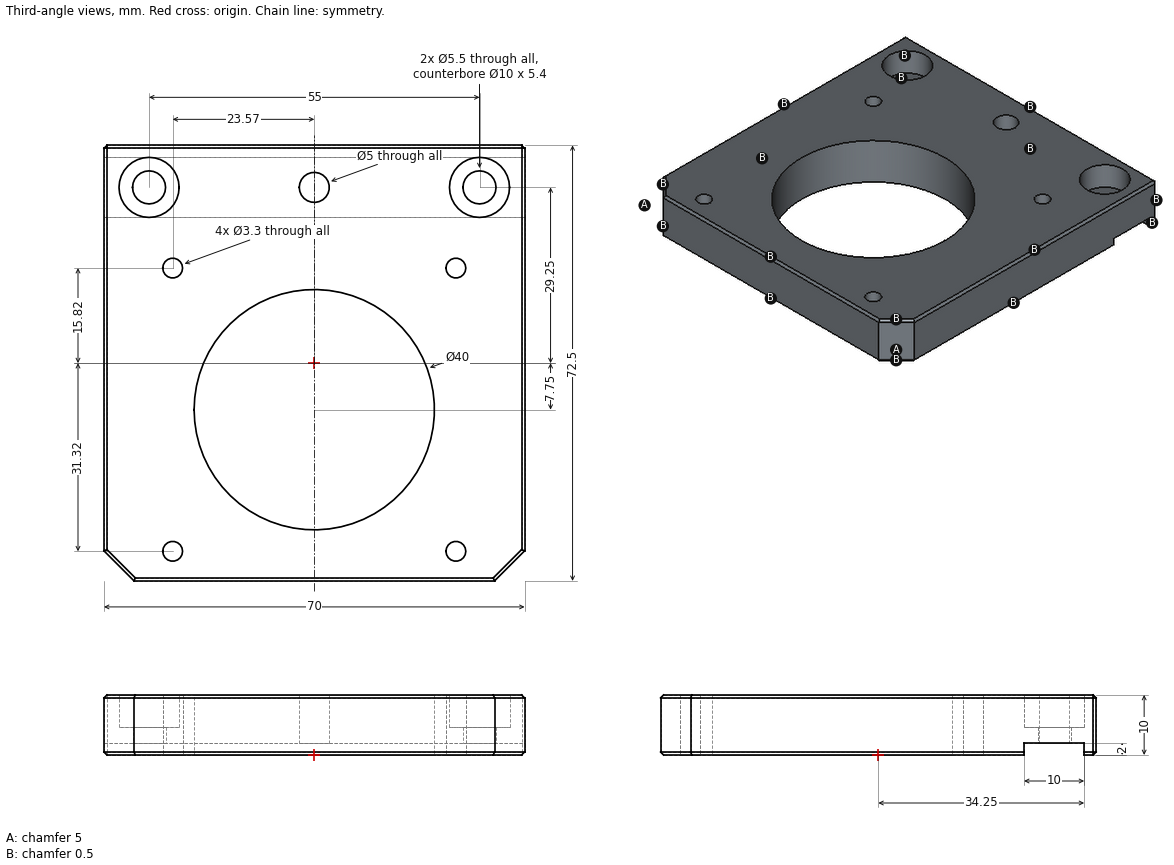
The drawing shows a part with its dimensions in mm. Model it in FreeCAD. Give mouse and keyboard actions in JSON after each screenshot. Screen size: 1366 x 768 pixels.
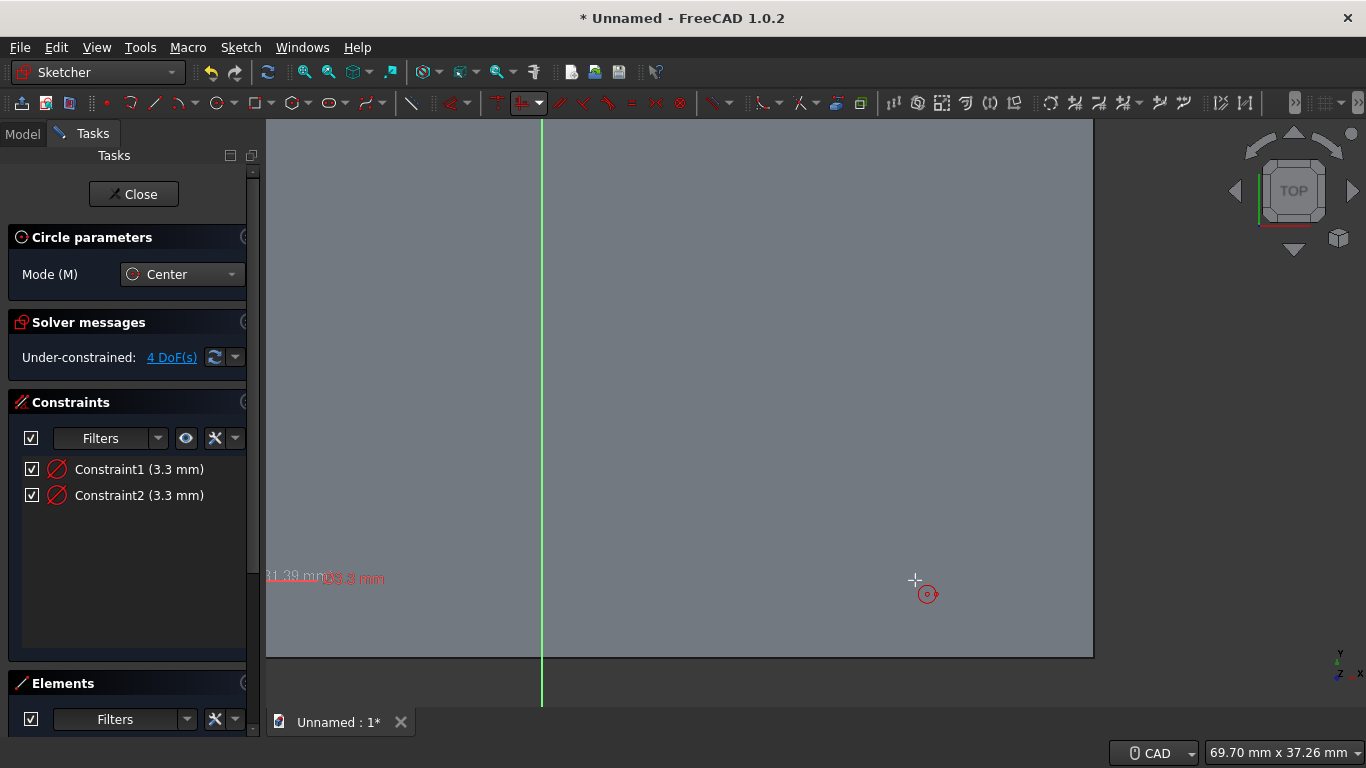
{"action": "left_click", "coordinate": [914, 580]}
{"action": "mouse_move", "coordinate": [932, 561]}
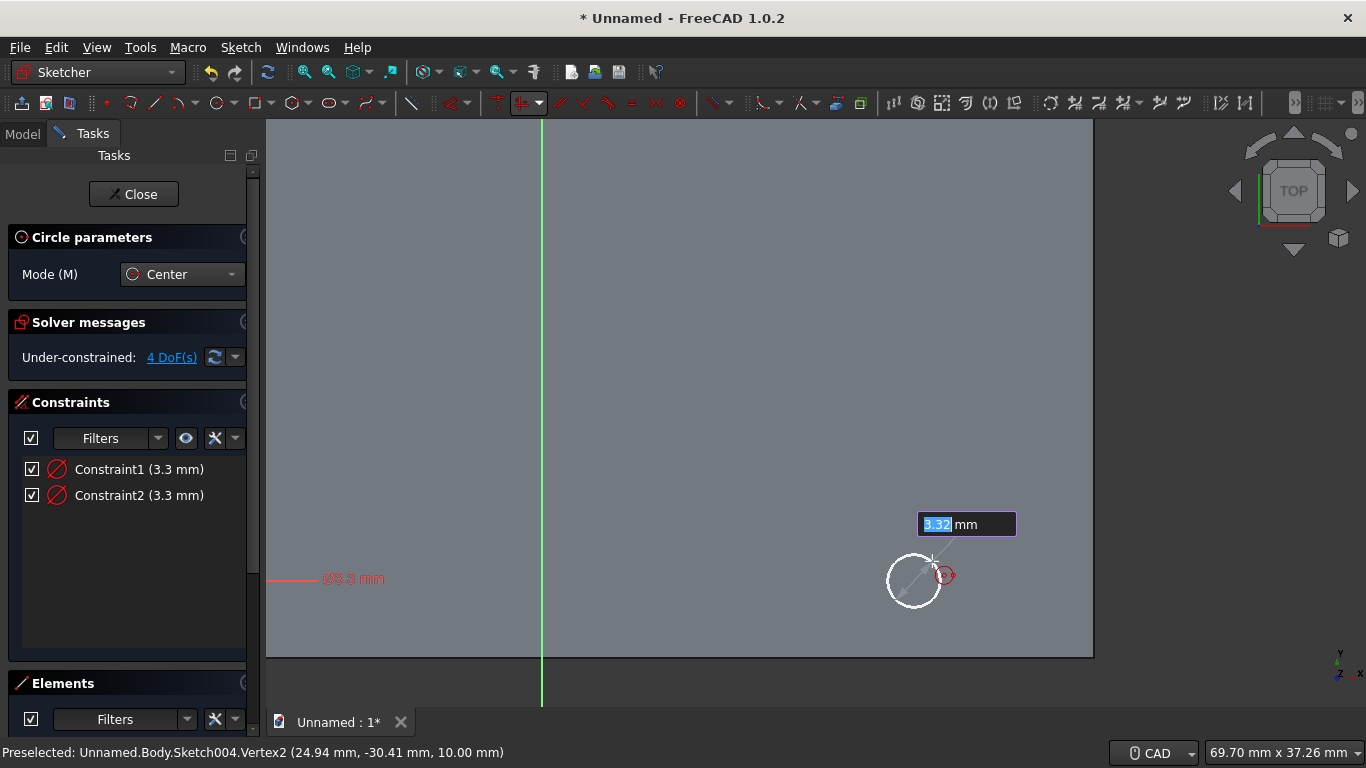
{"action": "type", "text": "3.3"}
{"action": "key", "text": "Return"}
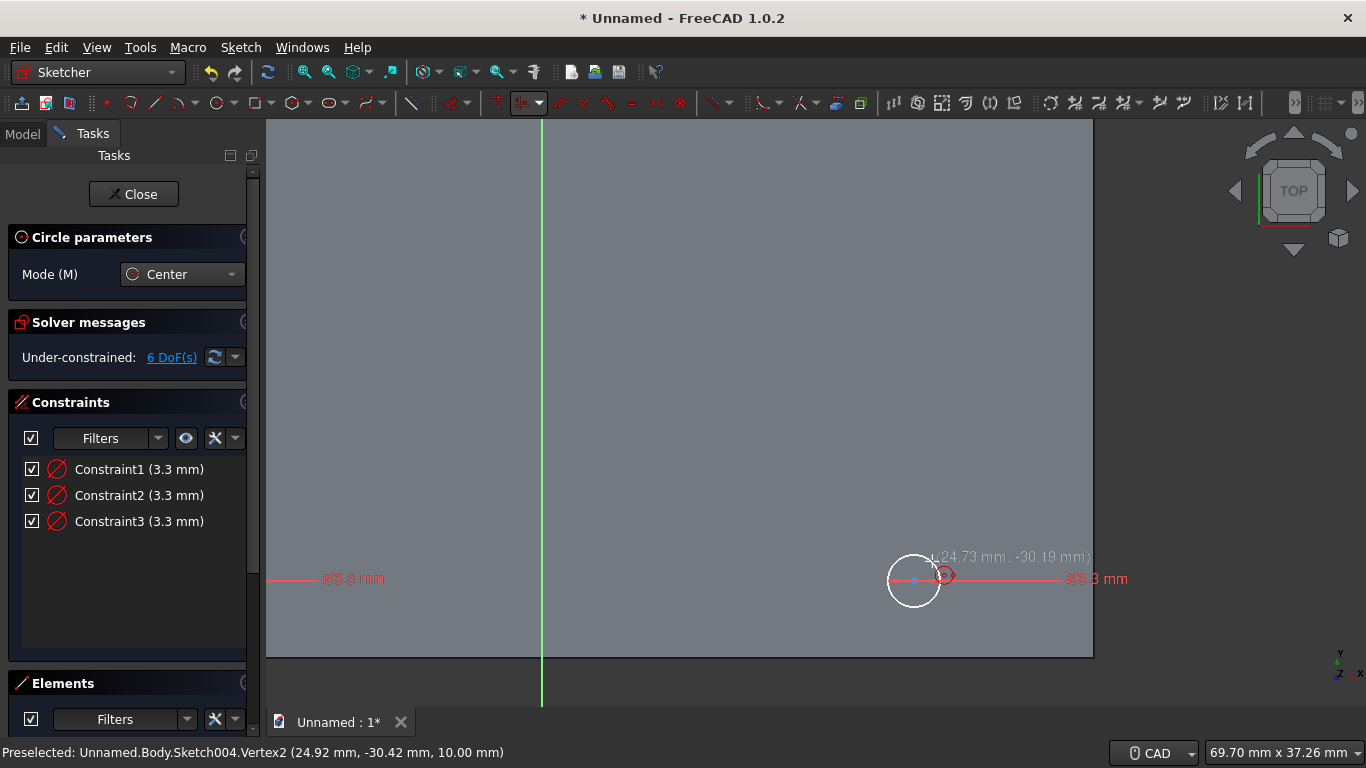
{"action": "scroll", "coordinate": [915, 580], "scroll_direction": "down", "scroll_amount": 4}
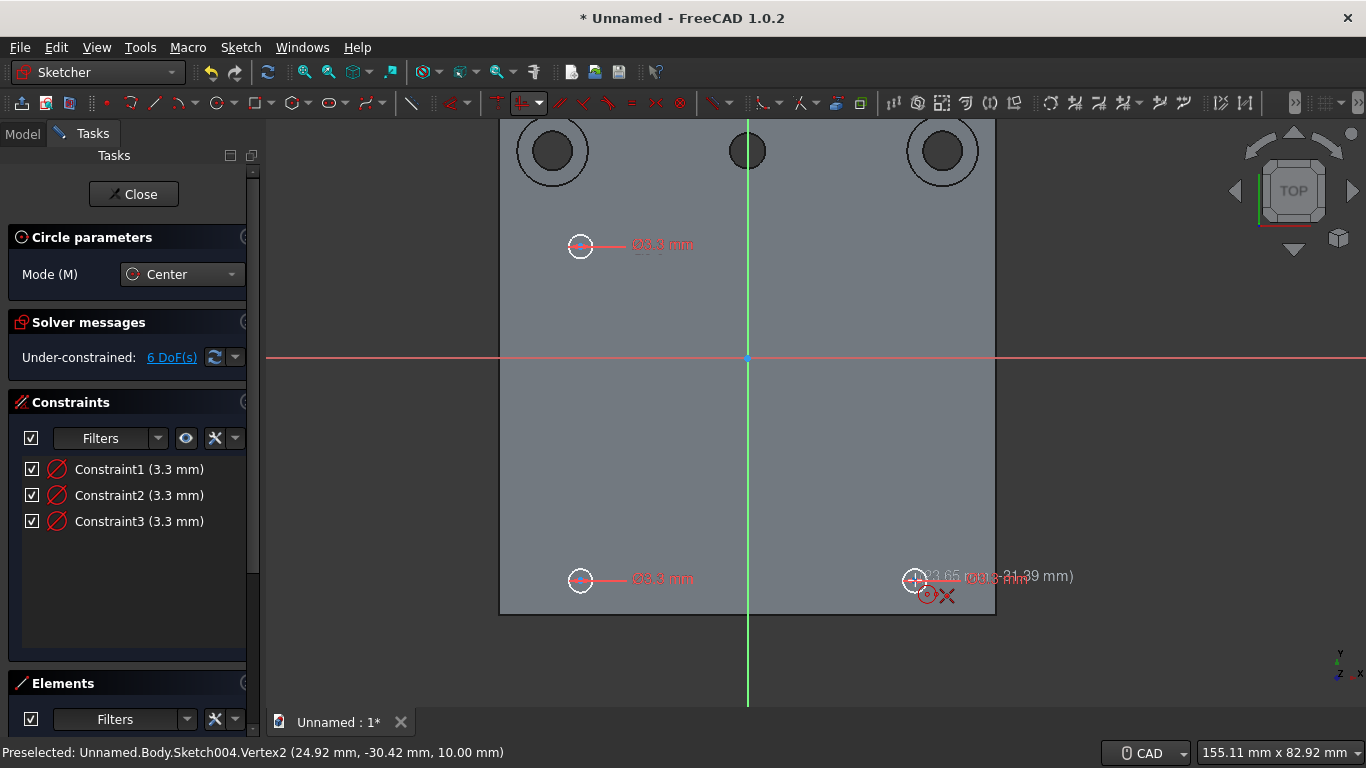
{"action": "scroll", "coordinate": [915, 246], "scroll_direction": "up", "scroll_amount": 4}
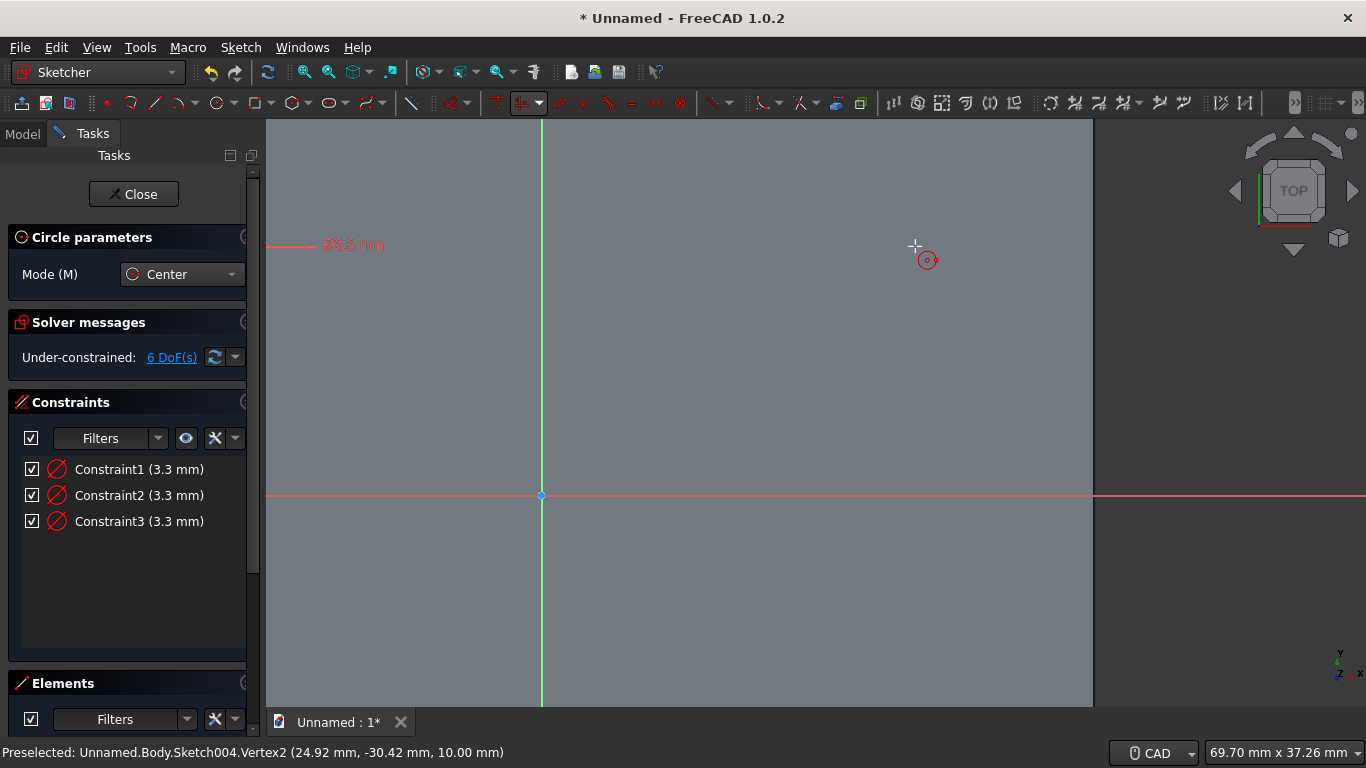
{"action": "left_click", "coordinate": [914, 246]}
{"action": "mouse_move", "coordinate": [932, 228]}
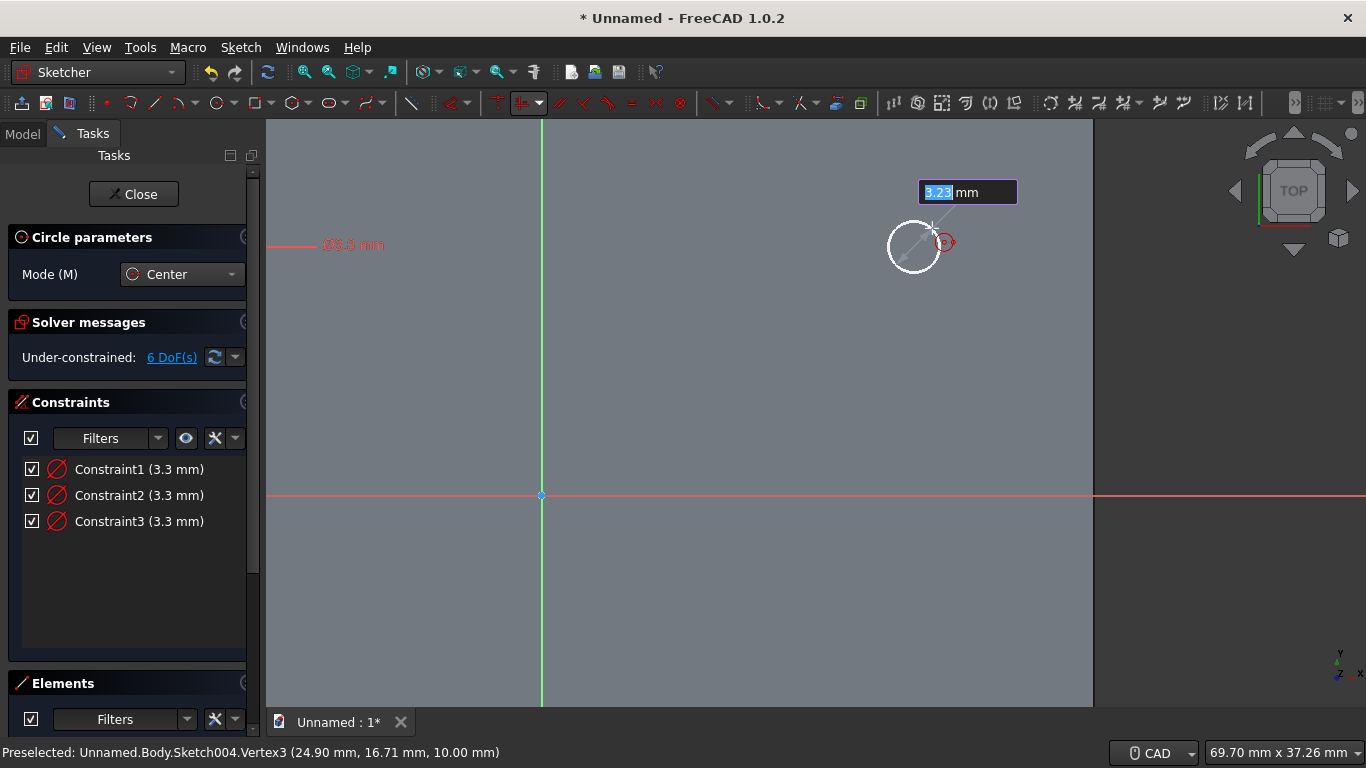
{"action": "type", "text": "3.3"}
{"action": "key", "text": "Return"}
{"action": "key", "text": "Escape"}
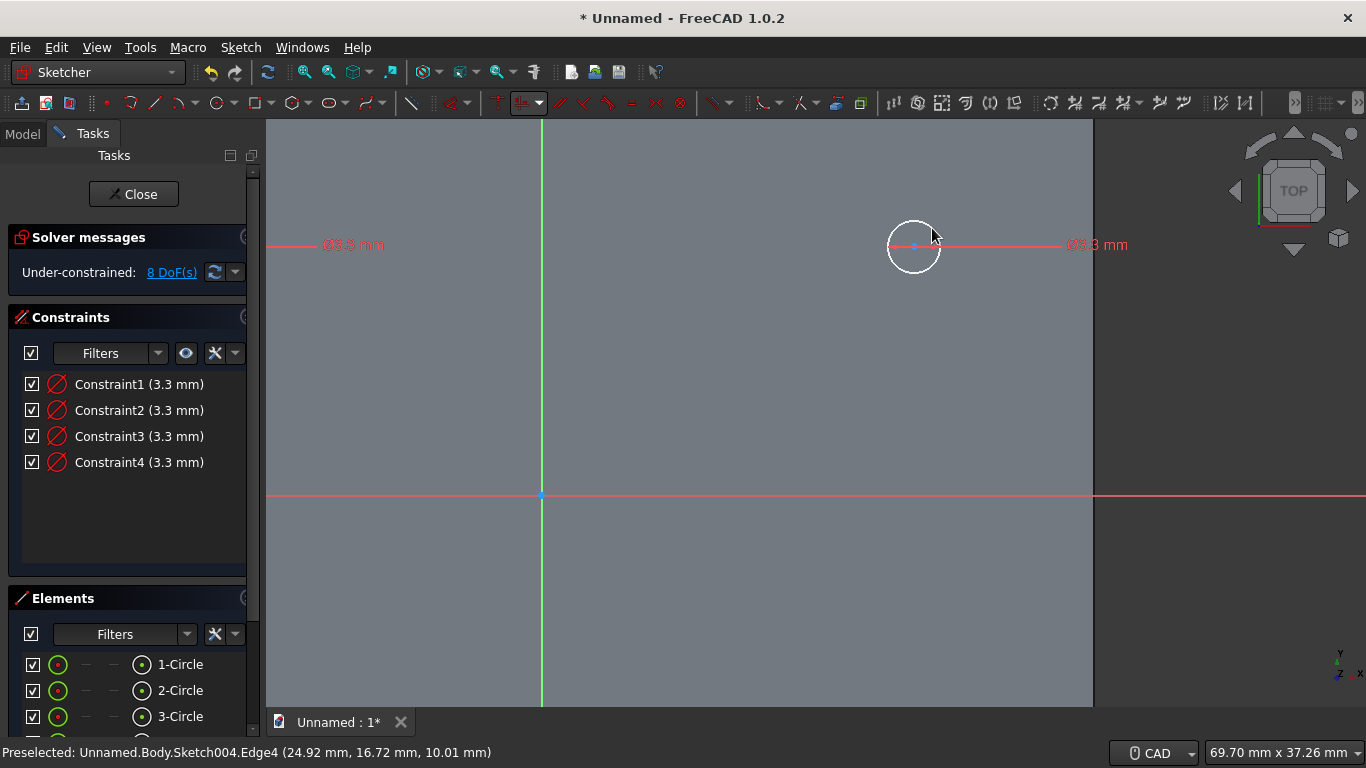
{"action": "scroll", "coordinate": [915, 246], "scroll_direction": "down", "scroll_amount": 4}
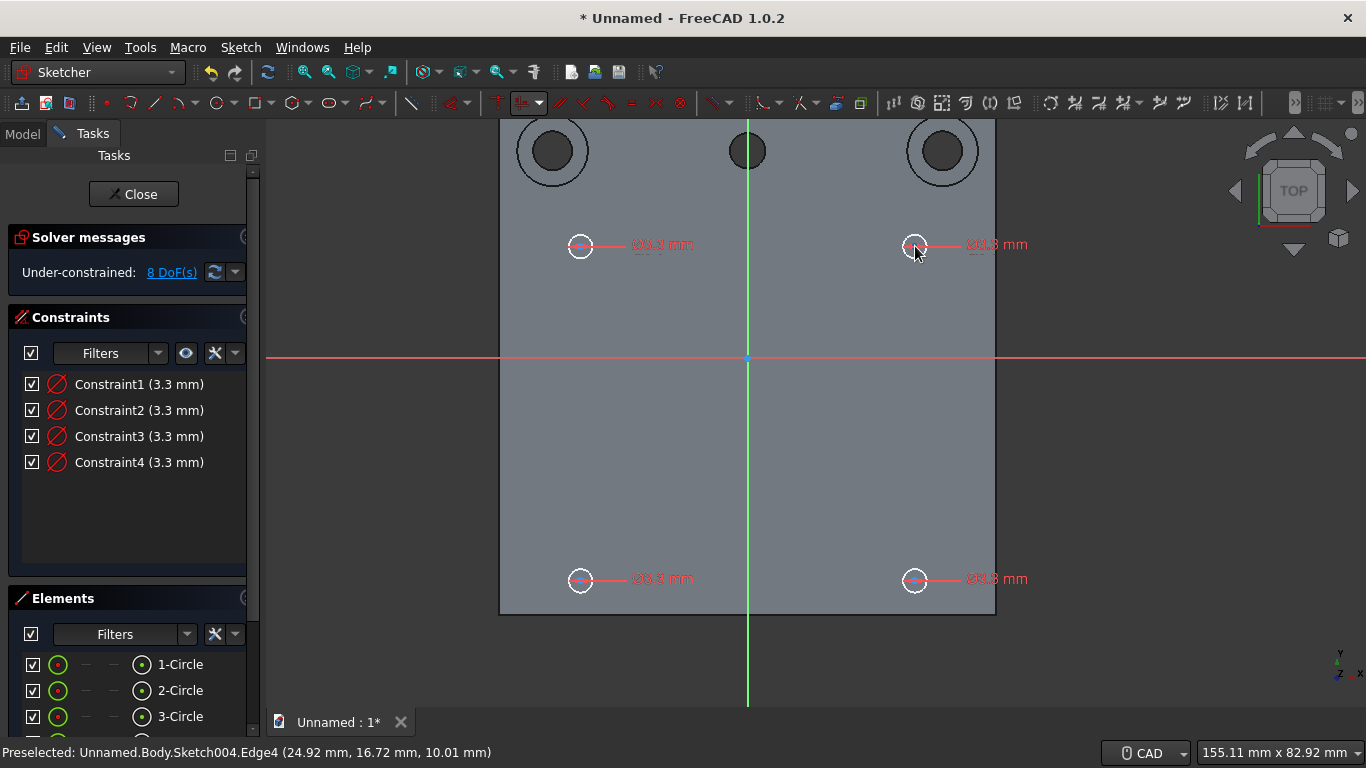
{"action": "left_click", "coordinate": [581, 581]}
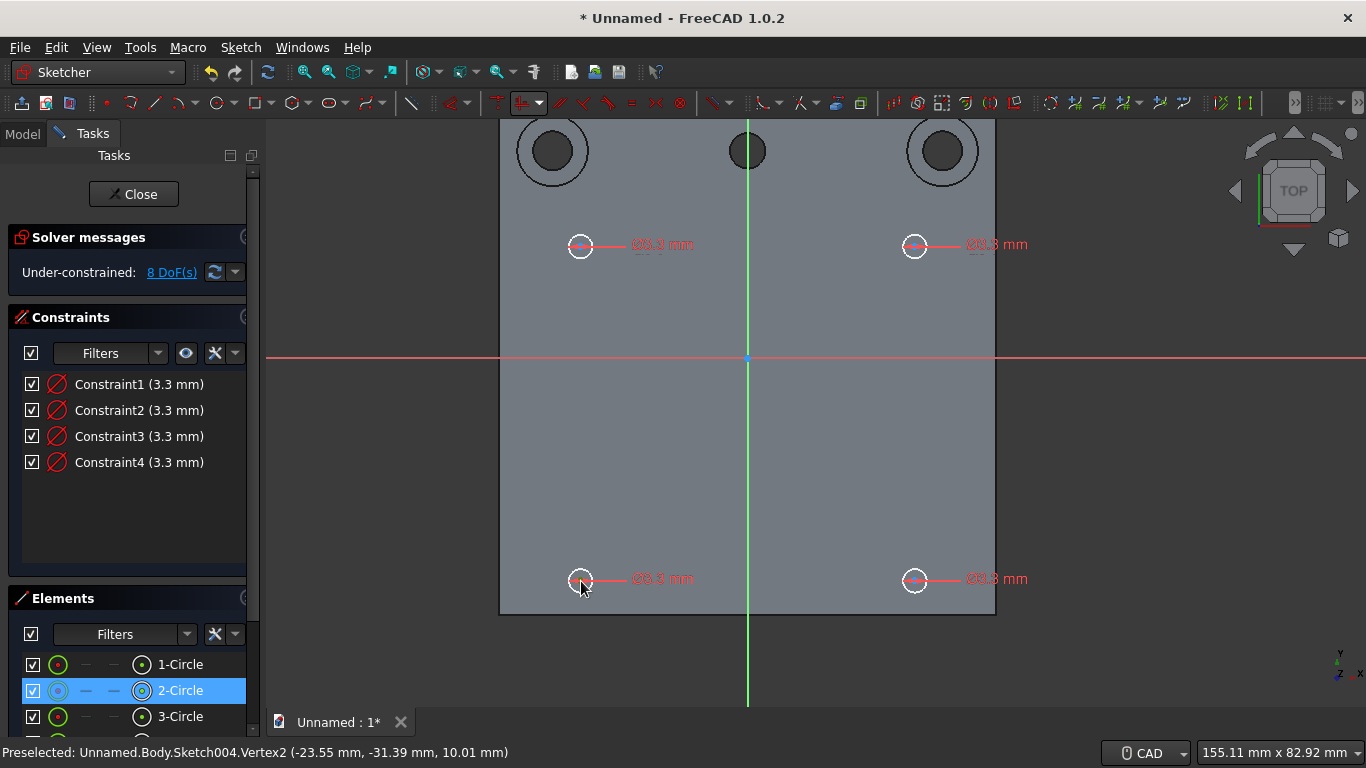
{"action": "left_click", "coordinate": [915, 581]}